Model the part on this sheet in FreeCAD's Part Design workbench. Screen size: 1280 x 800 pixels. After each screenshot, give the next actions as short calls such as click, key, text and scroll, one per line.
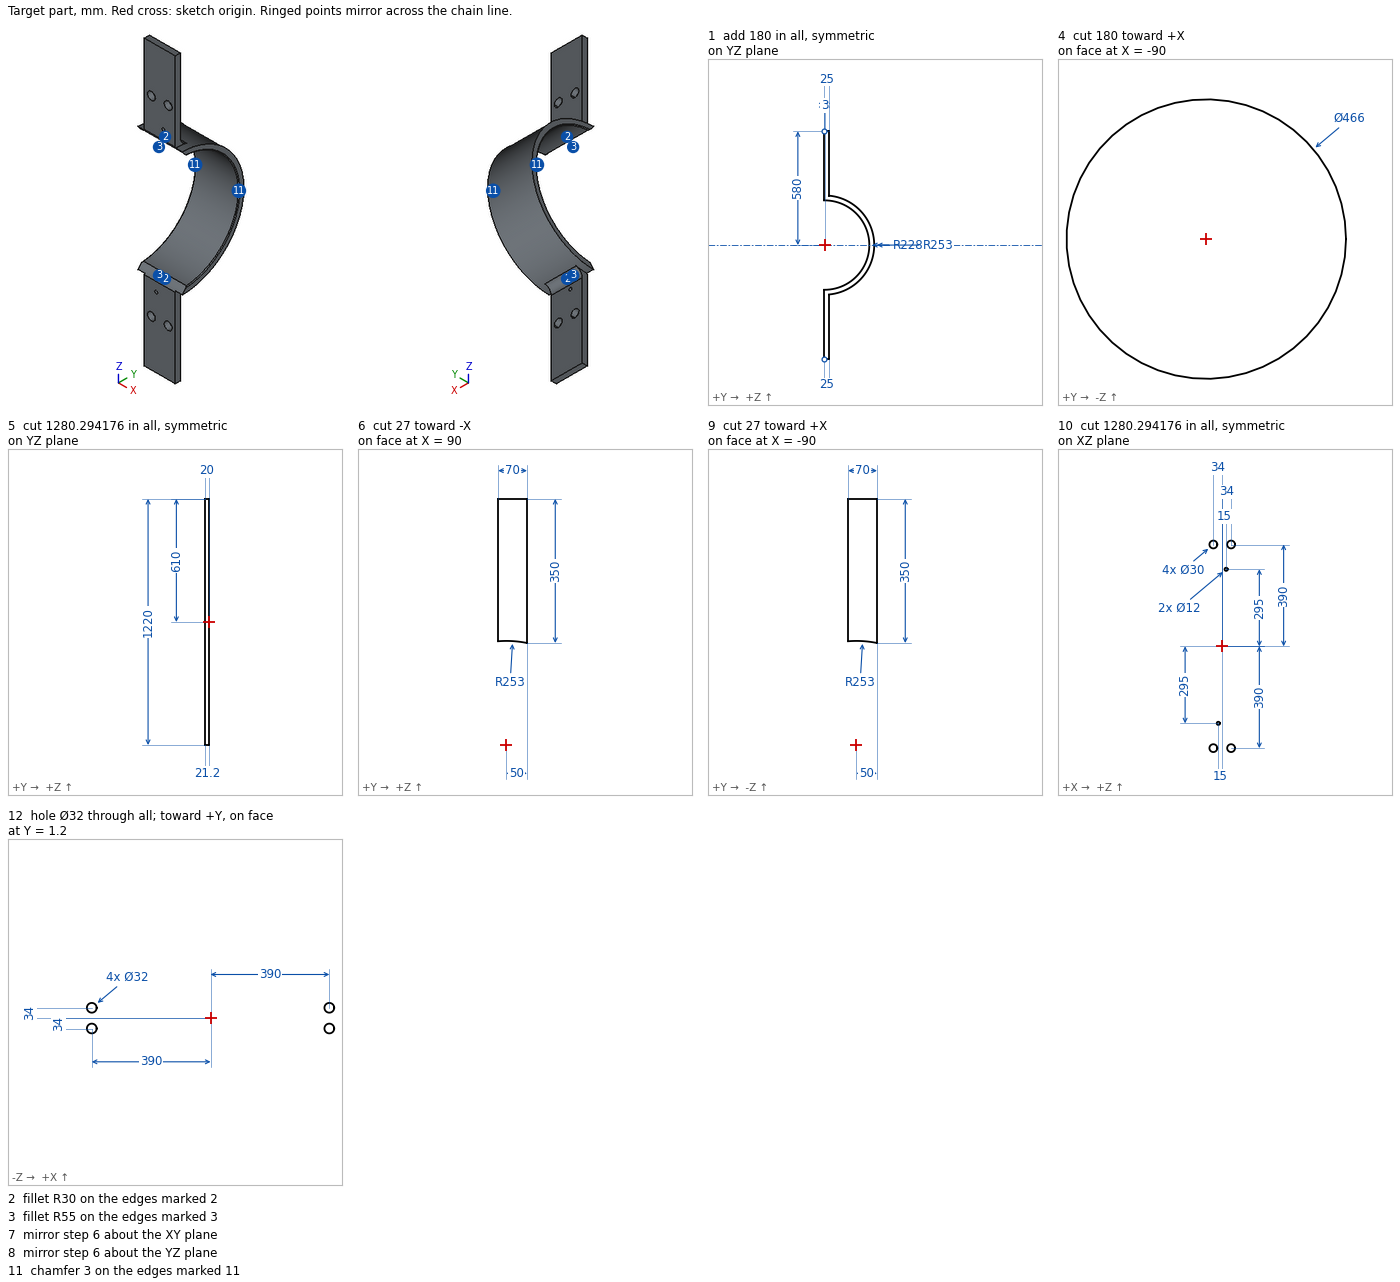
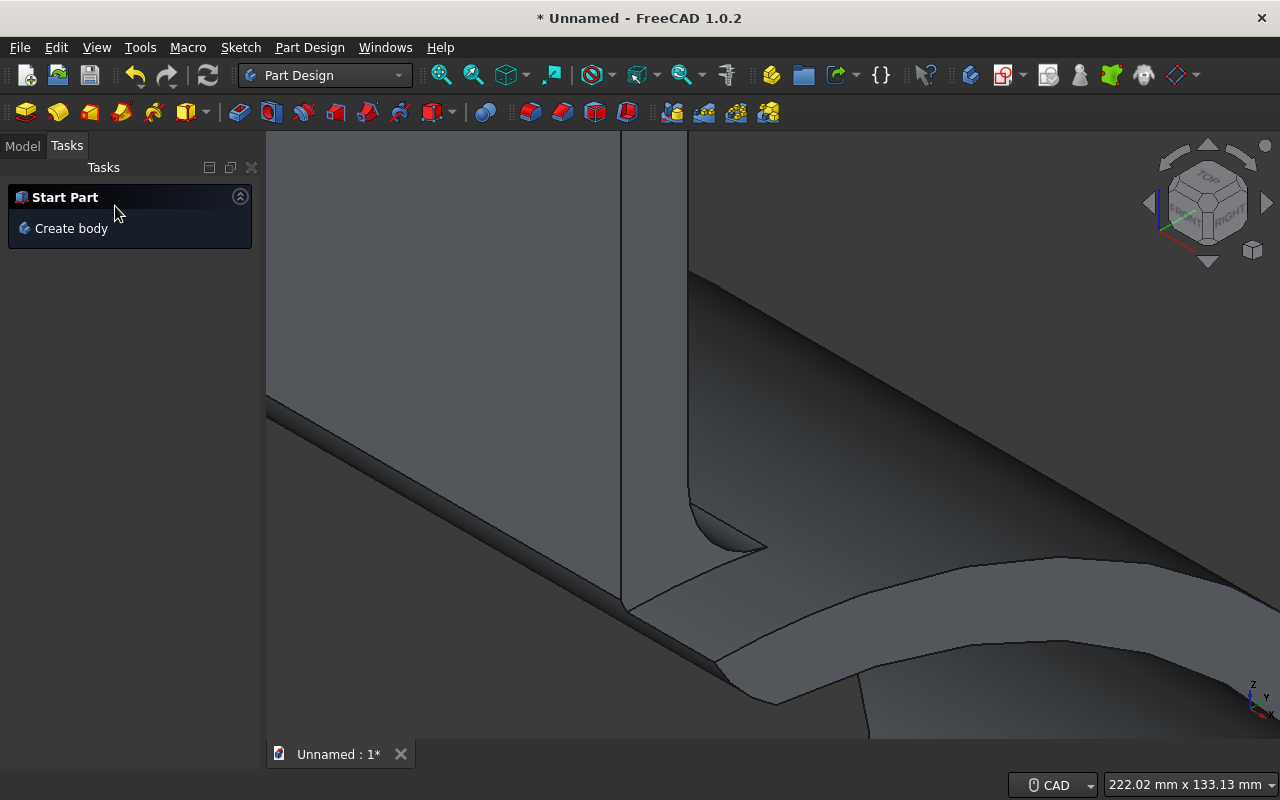
click(442, 76)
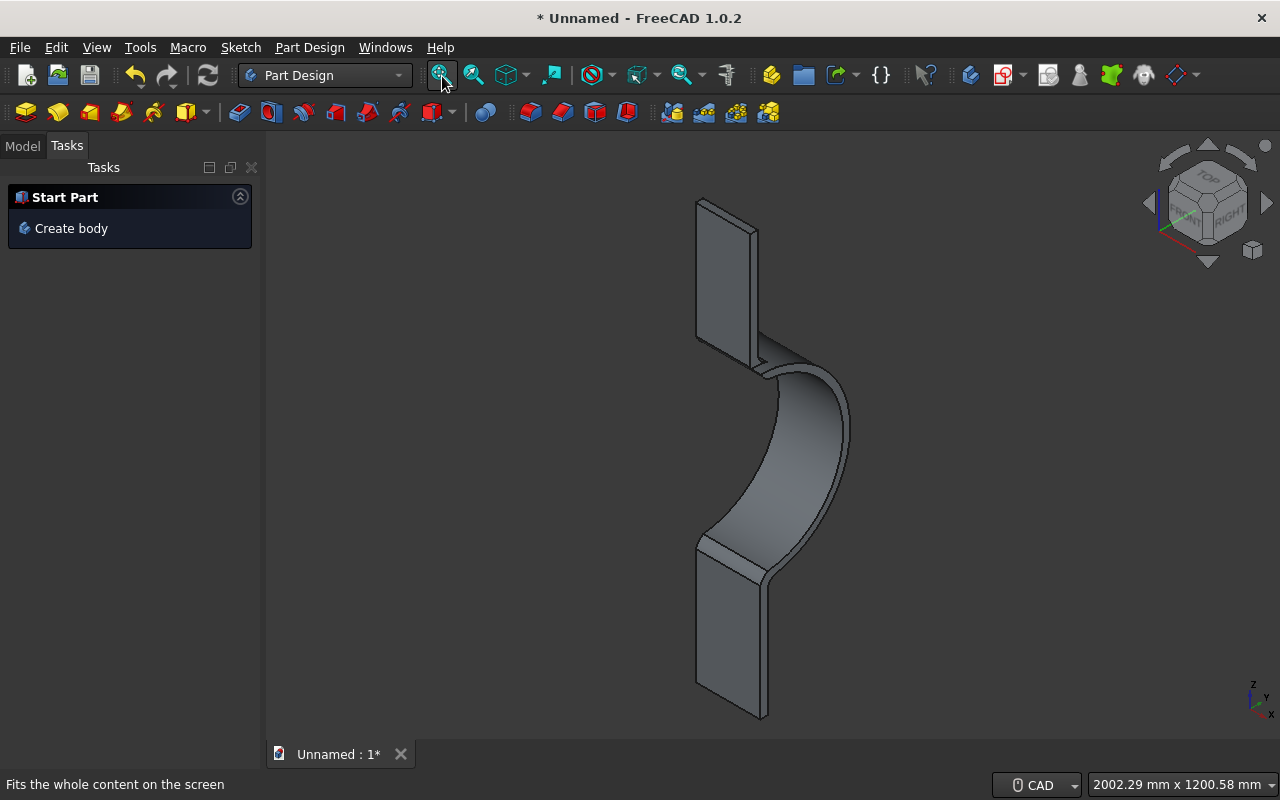
click(23, 145)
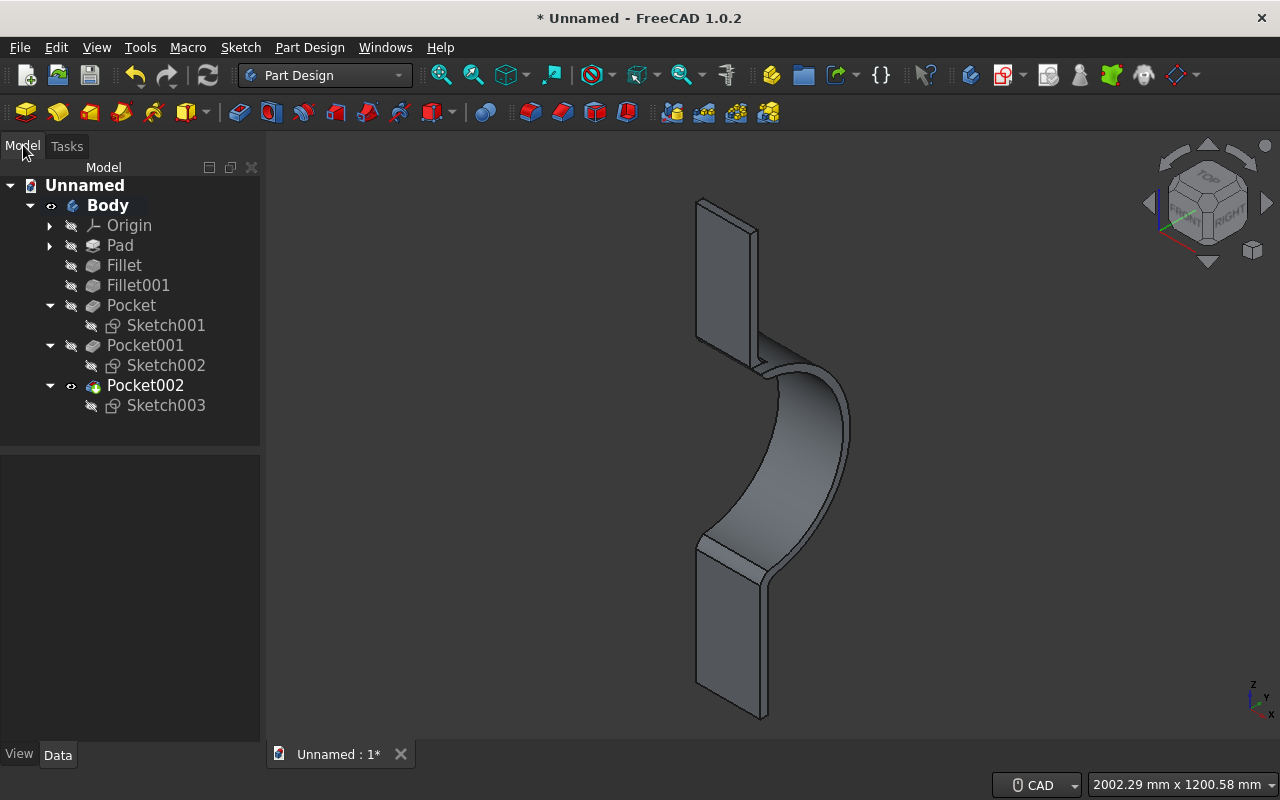
click(116, 386)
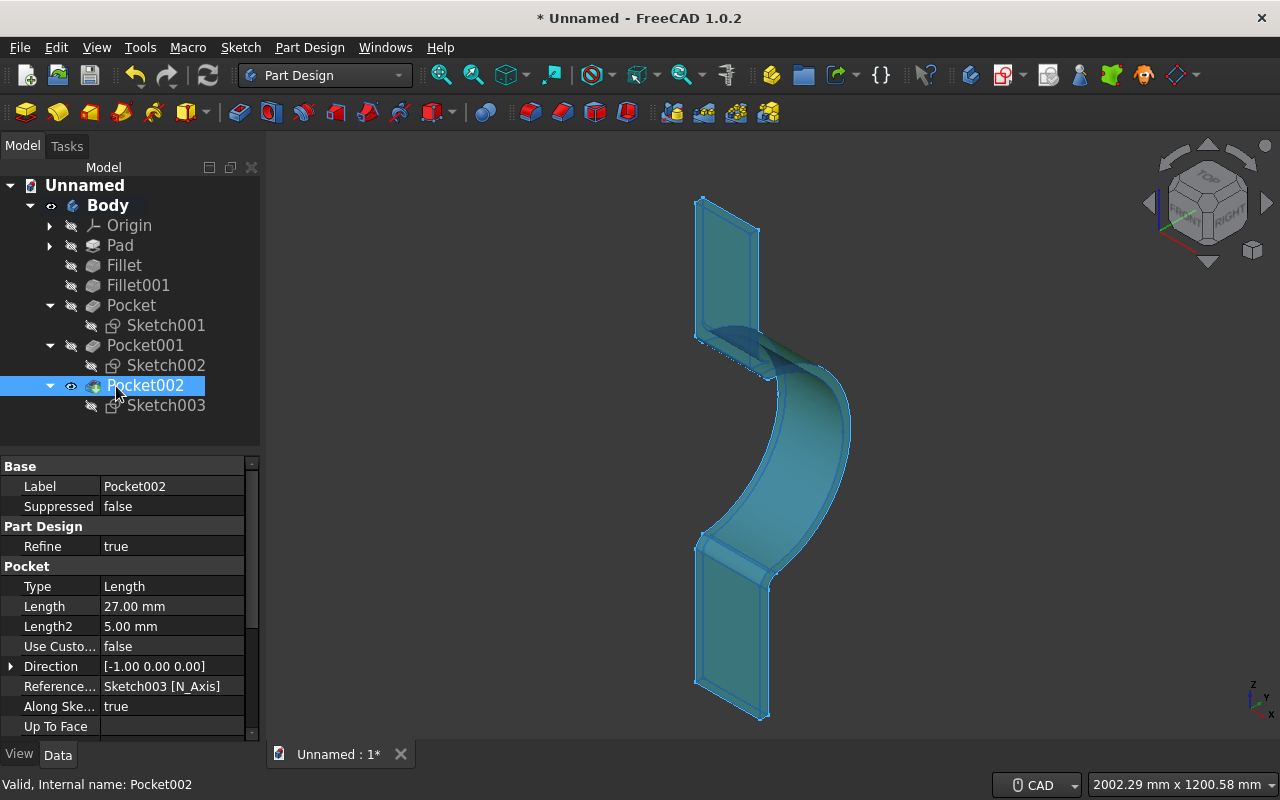
click(672, 112)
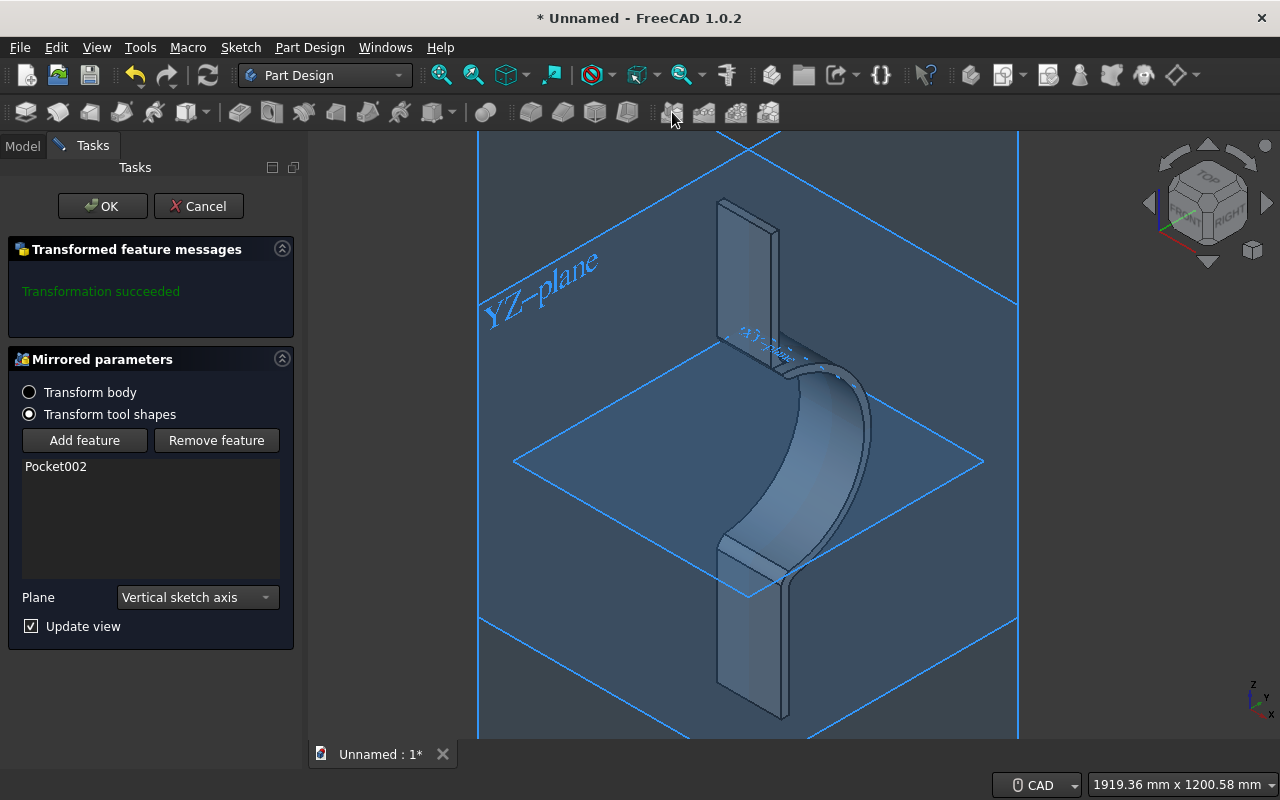
click(198, 598)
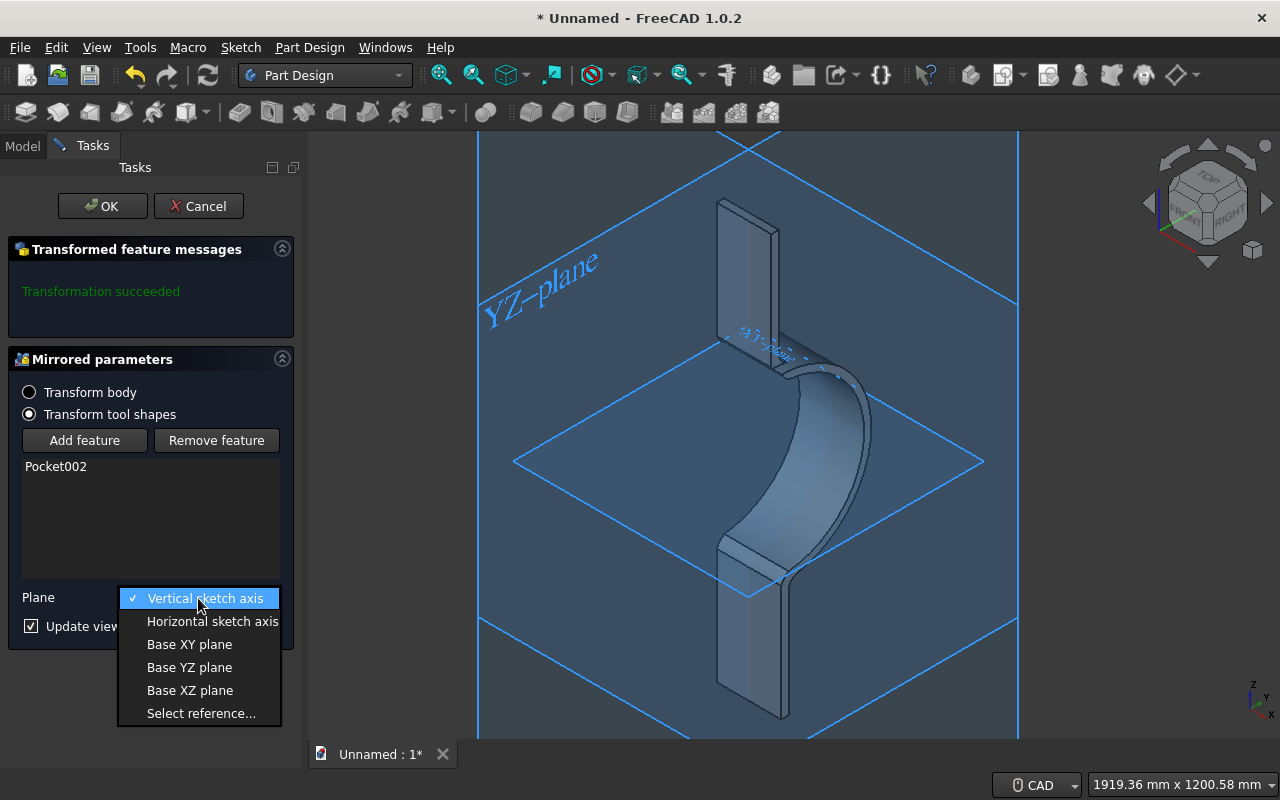
click(198, 644)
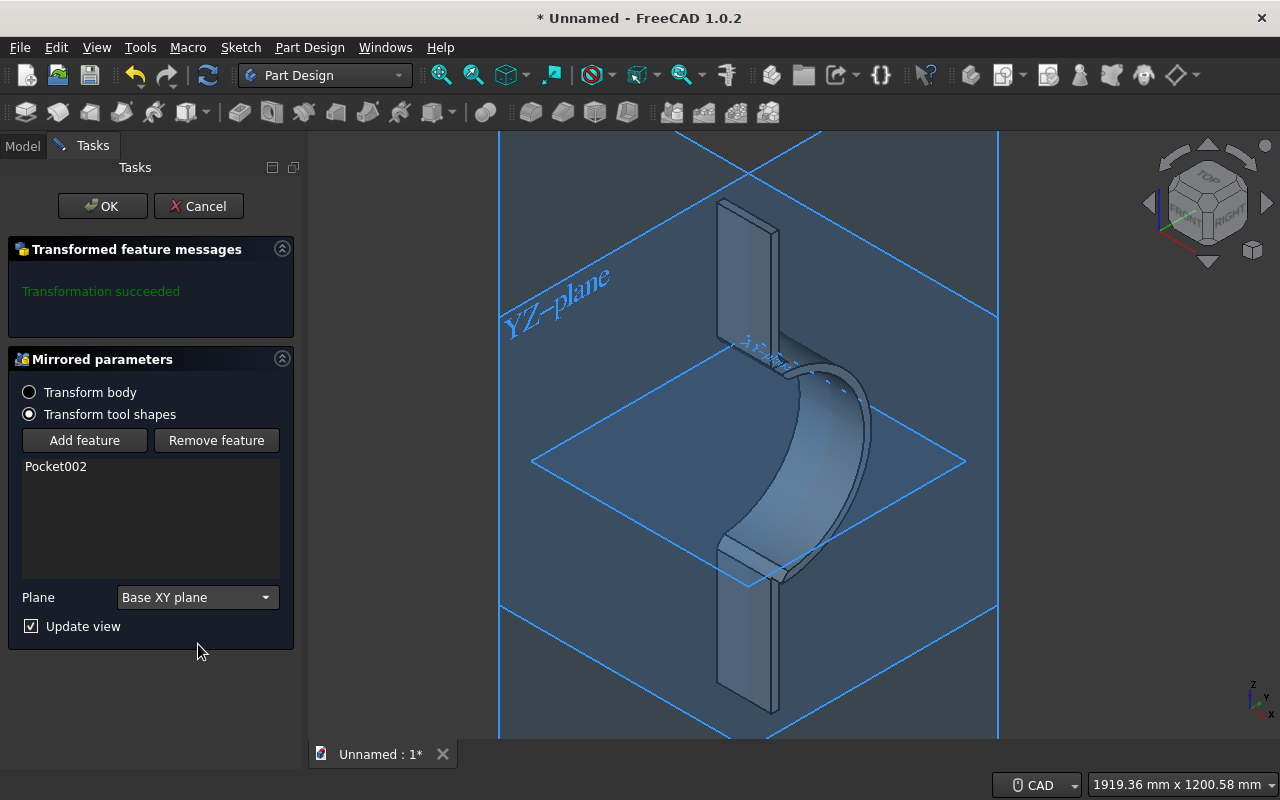
click(103, 206)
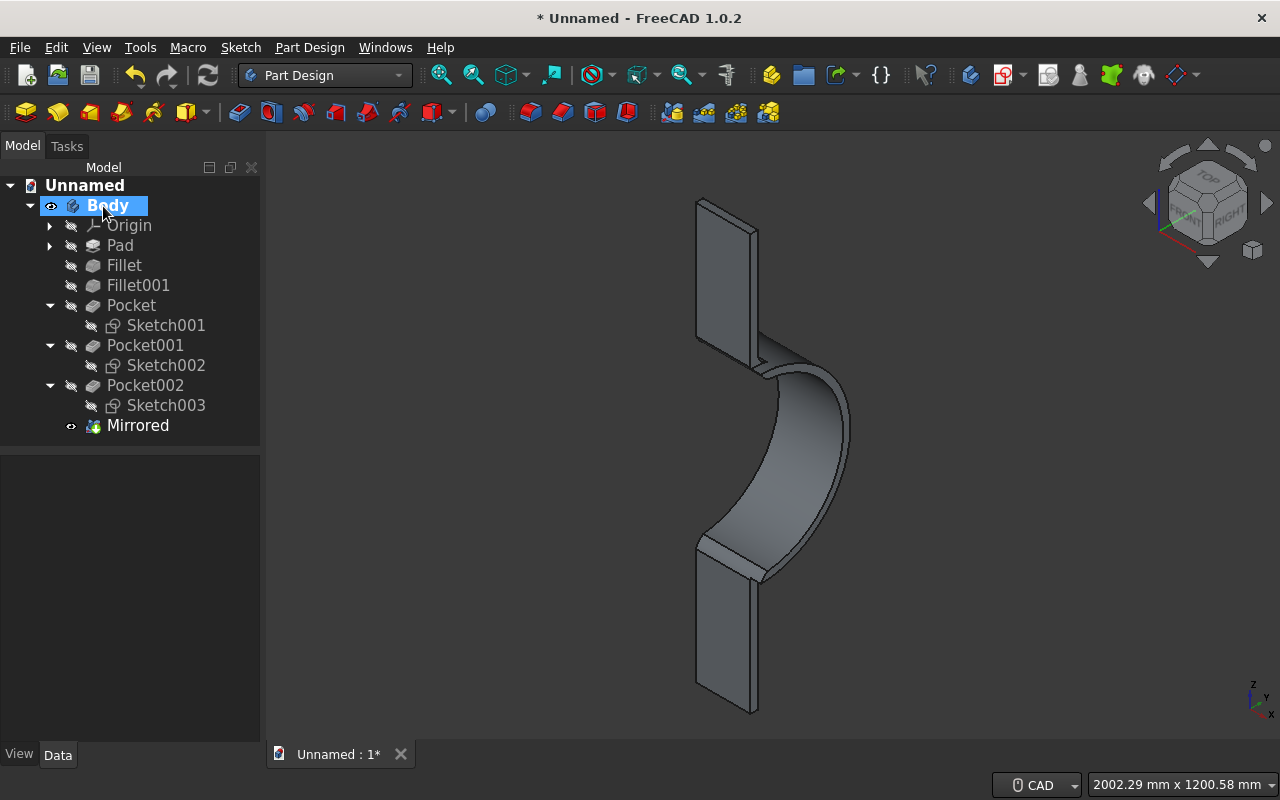
click(116, 386)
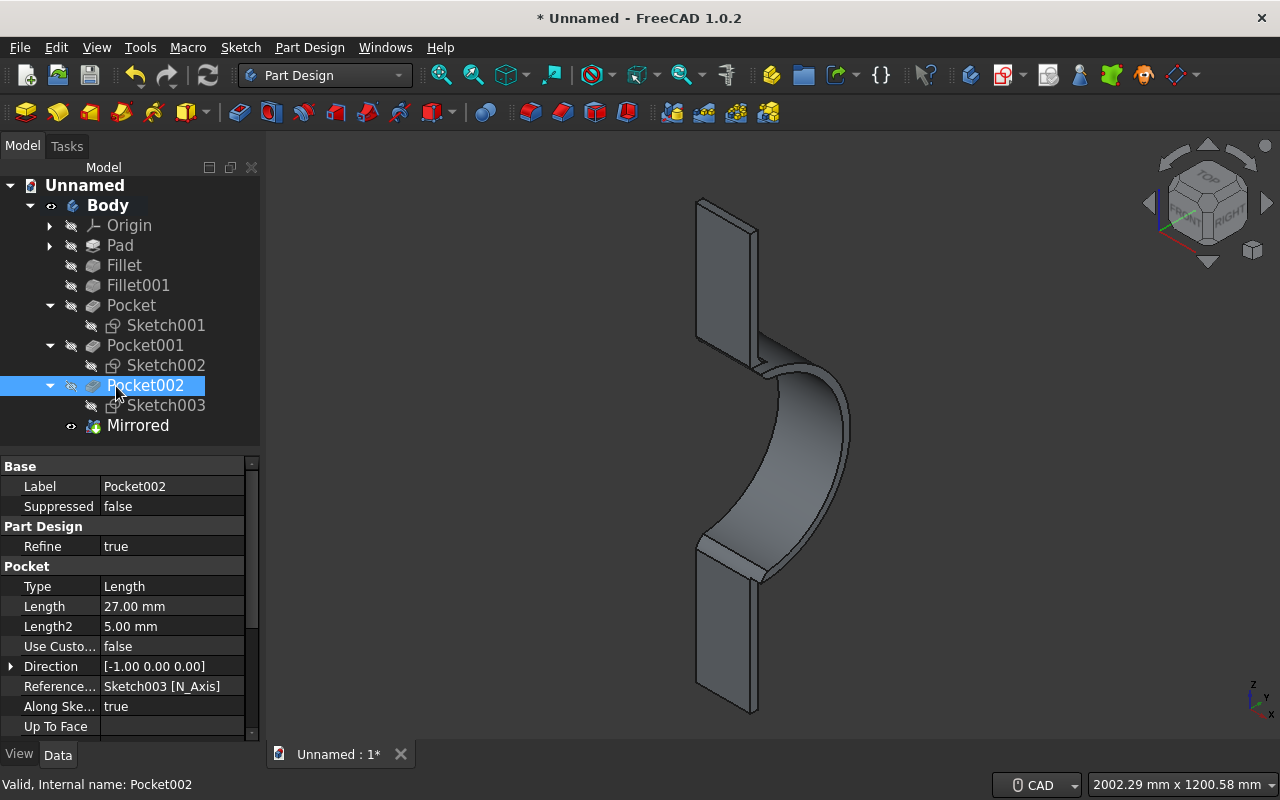
click(672, 112)